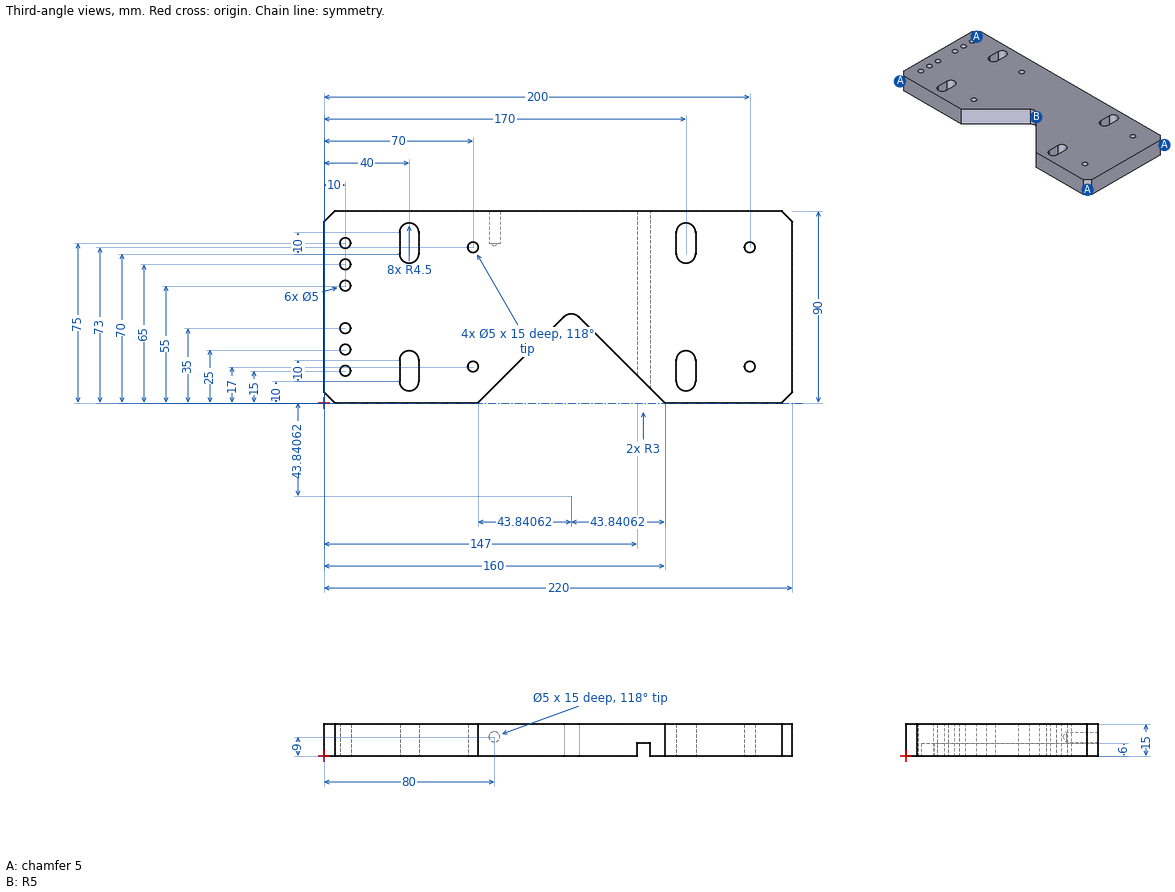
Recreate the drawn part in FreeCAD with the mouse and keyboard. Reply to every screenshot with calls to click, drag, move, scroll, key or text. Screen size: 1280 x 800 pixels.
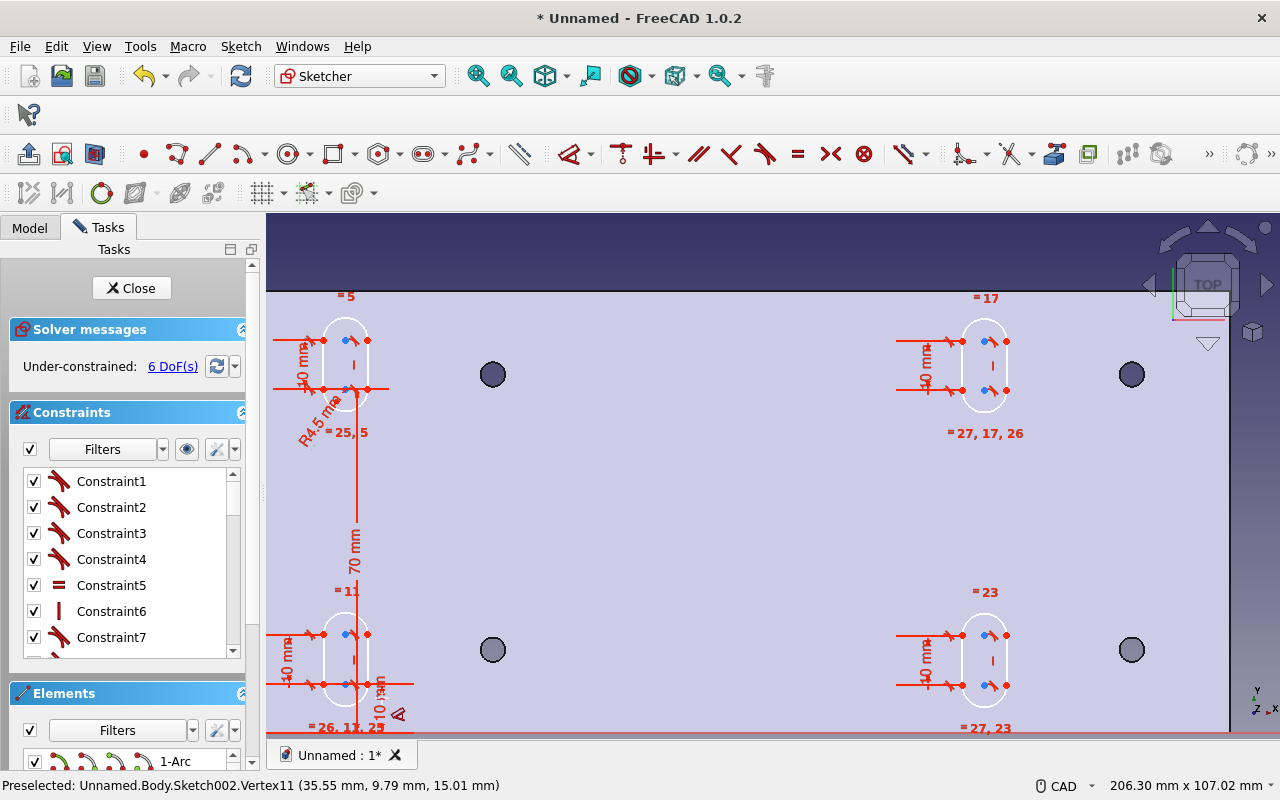
click(962, 390)
click(996, 551)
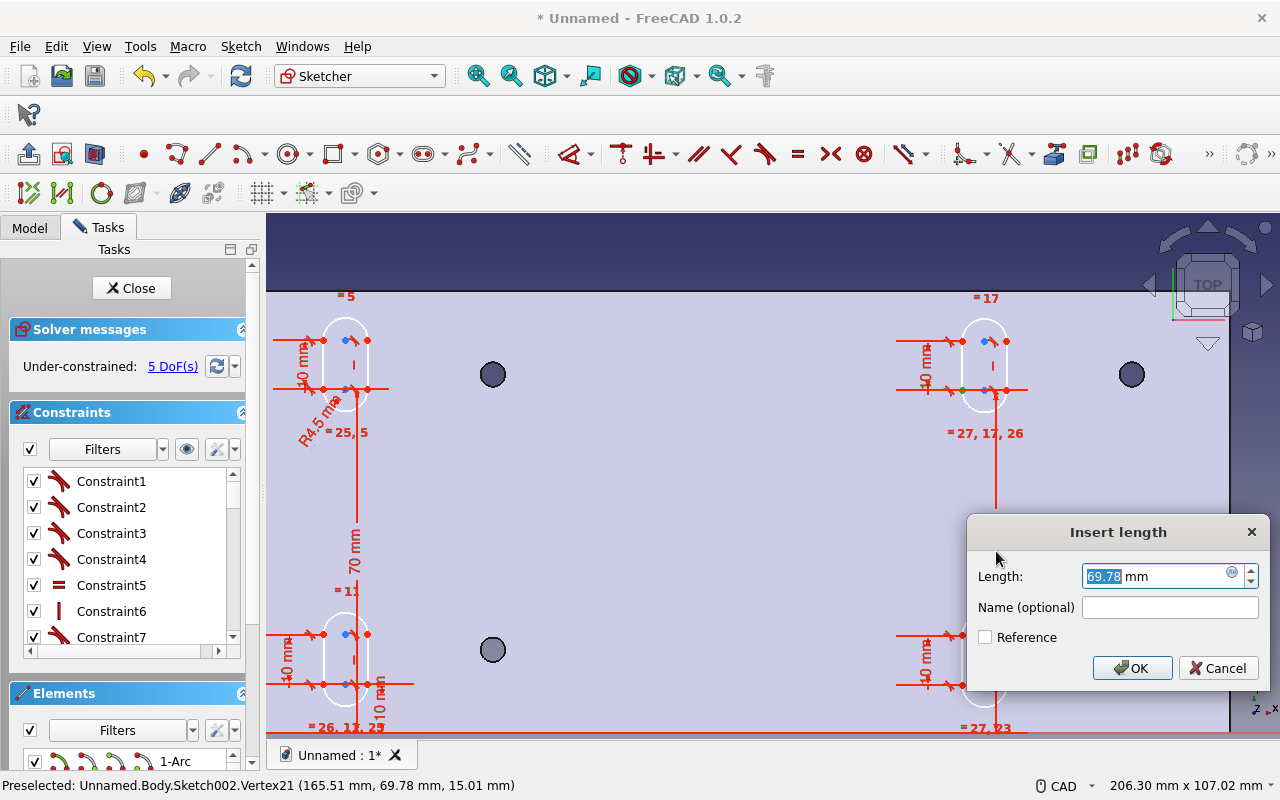
text(70)
key(Return)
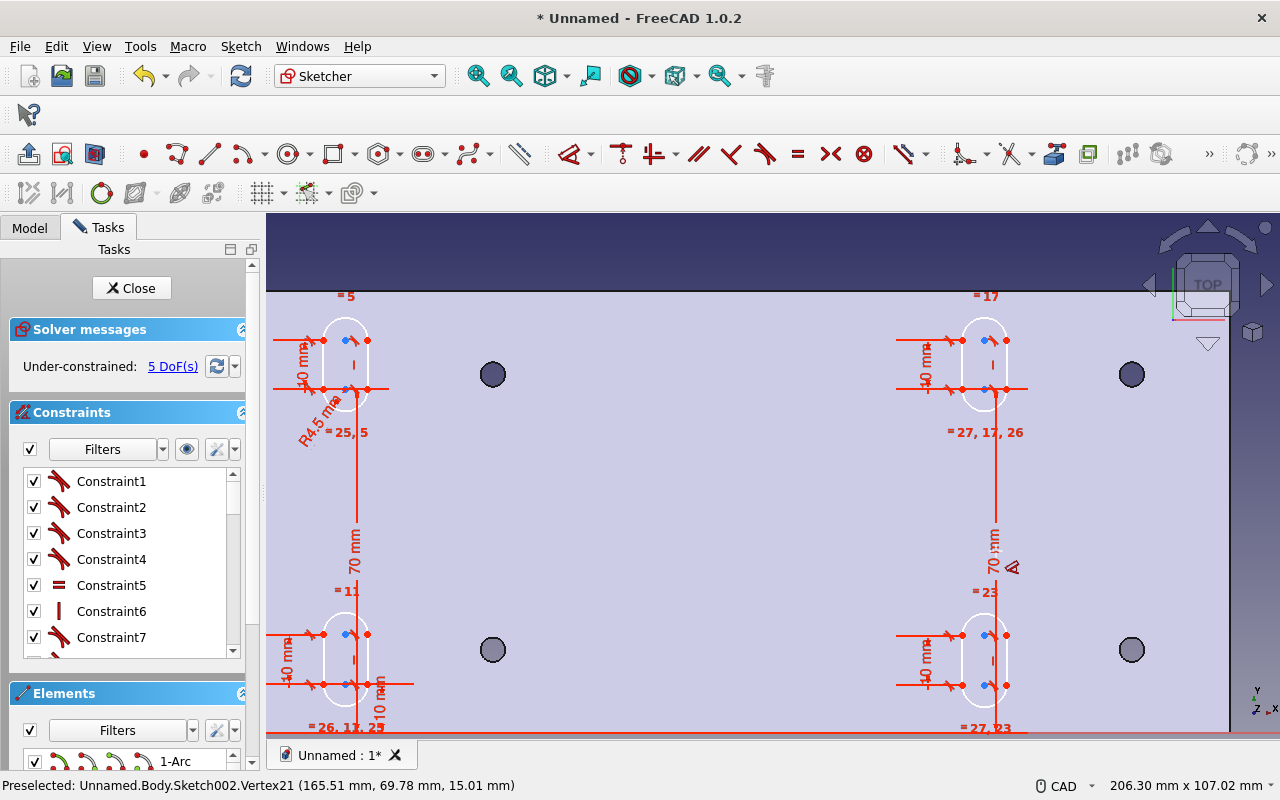
click(962, 685)
click(1020, 698)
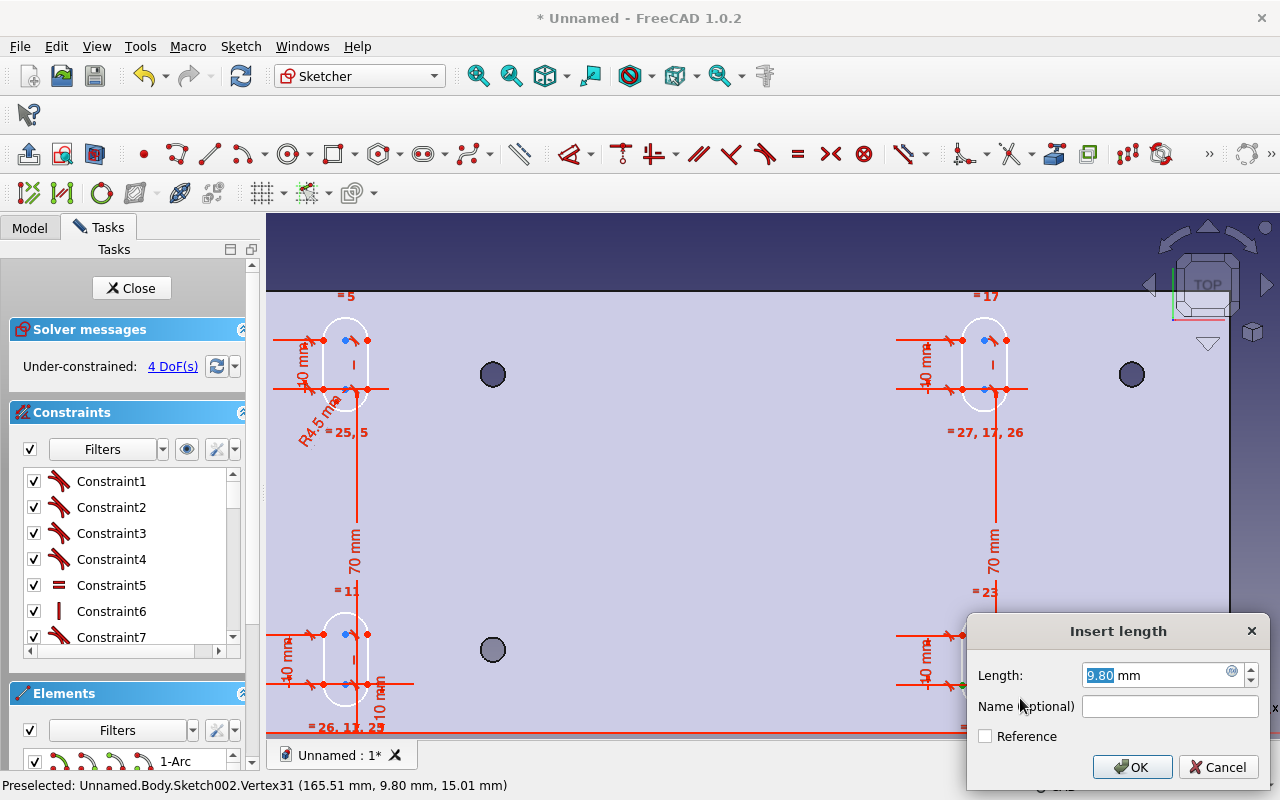
text(10)
key(Return)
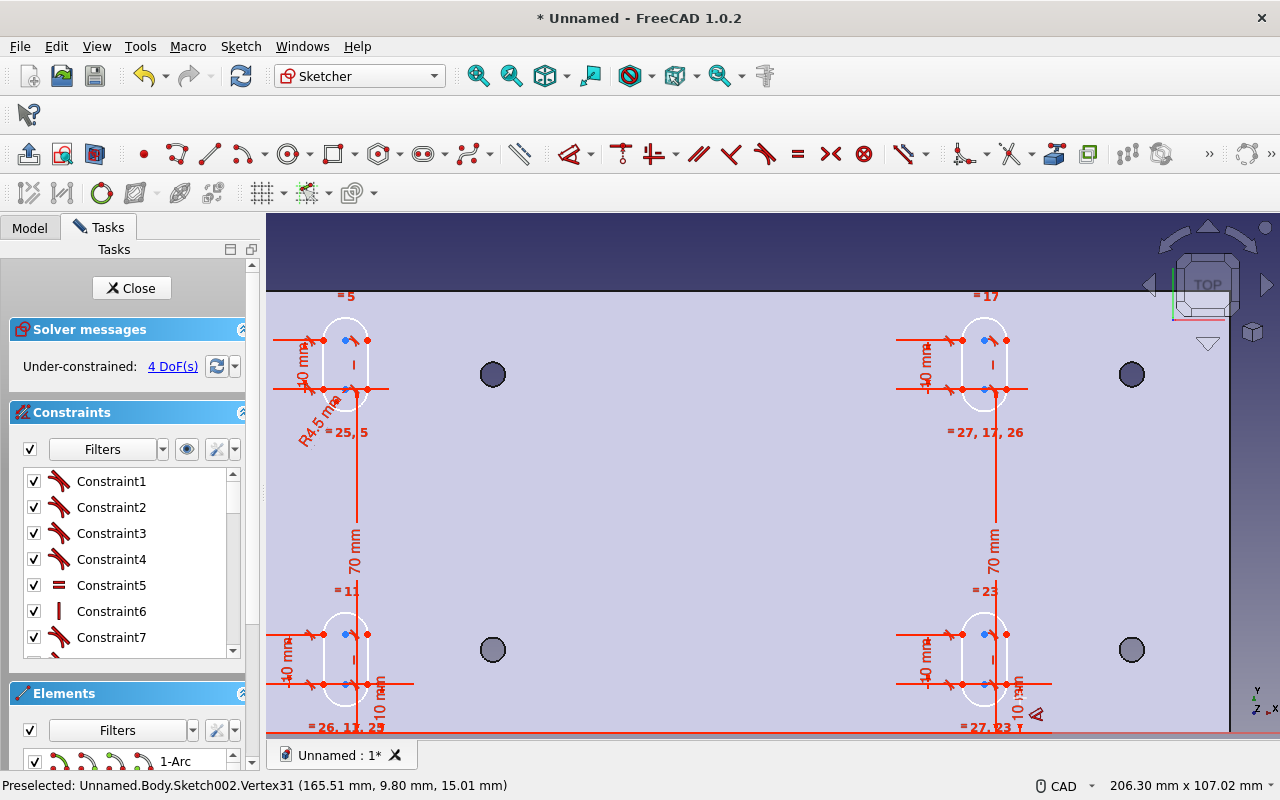
click(346, 389)
click(308, 331)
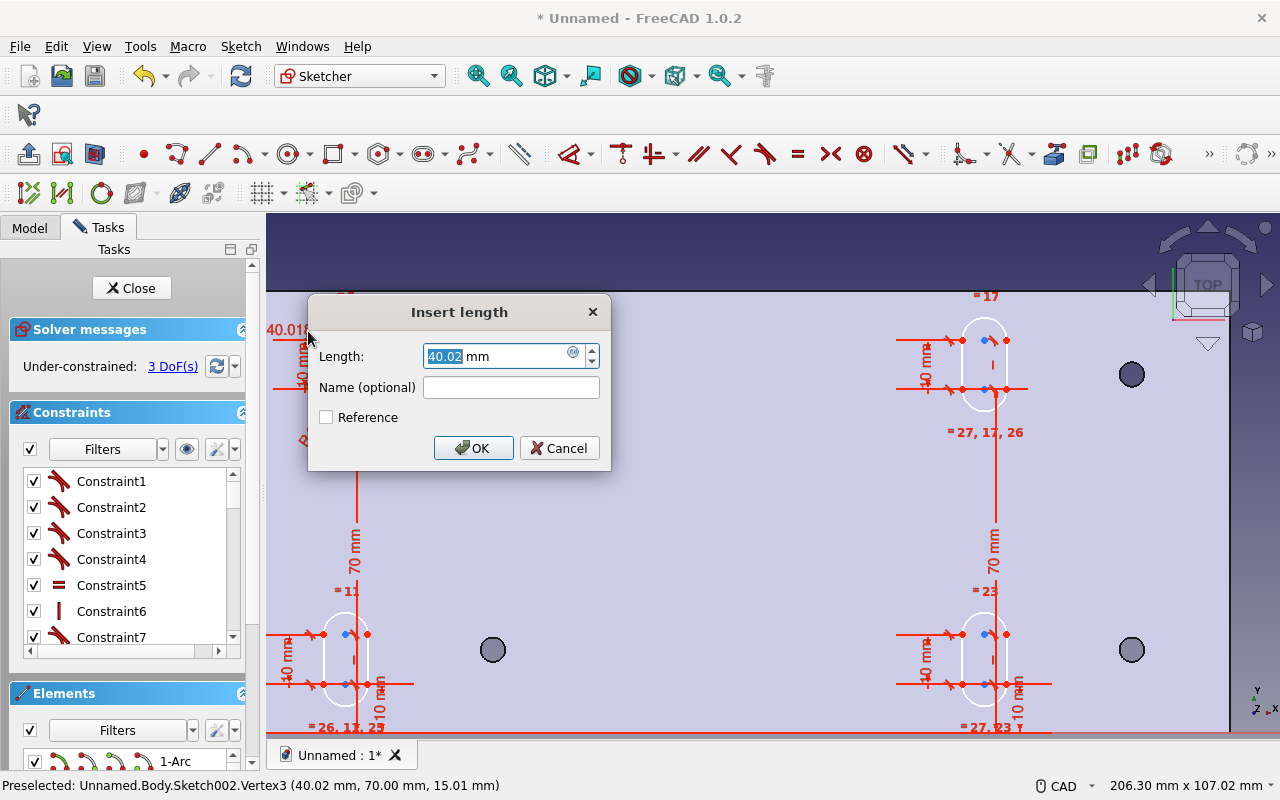
text(40)
key(Return)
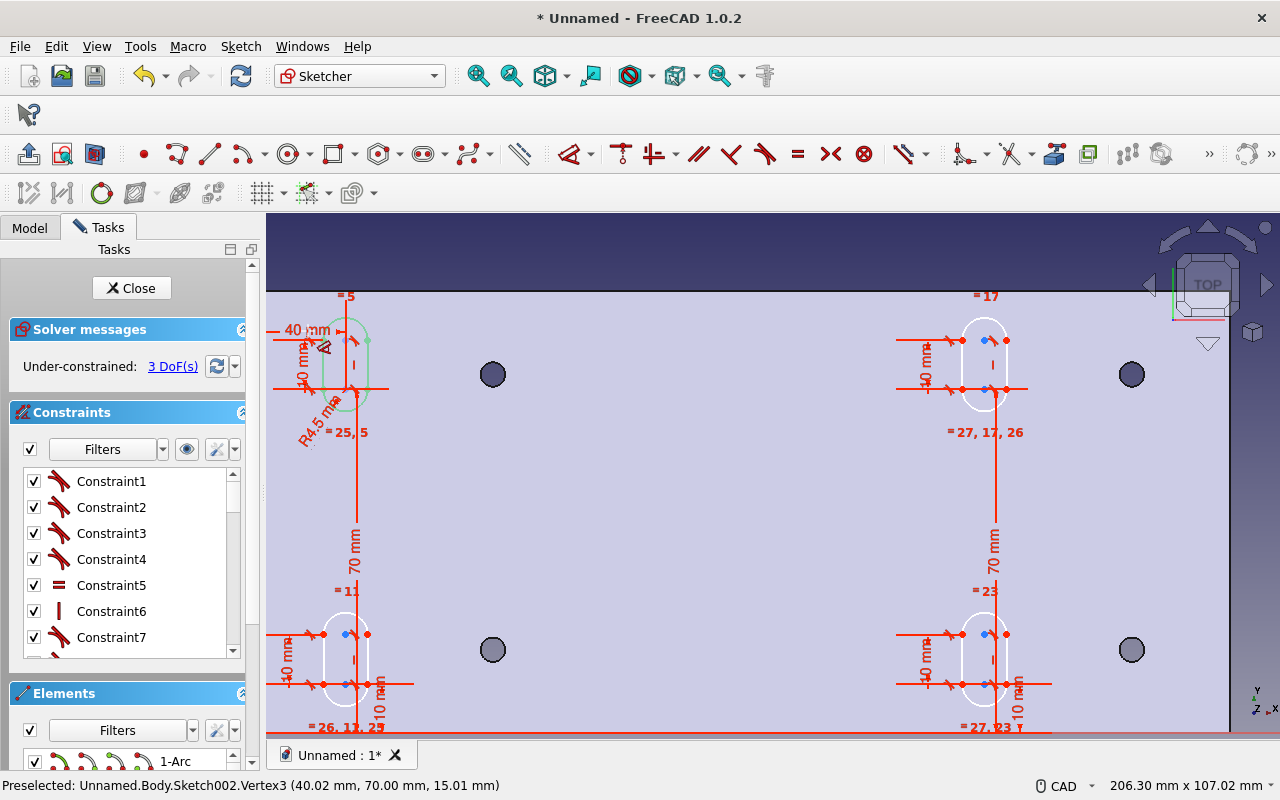
click(346, 684)
click(308, 626)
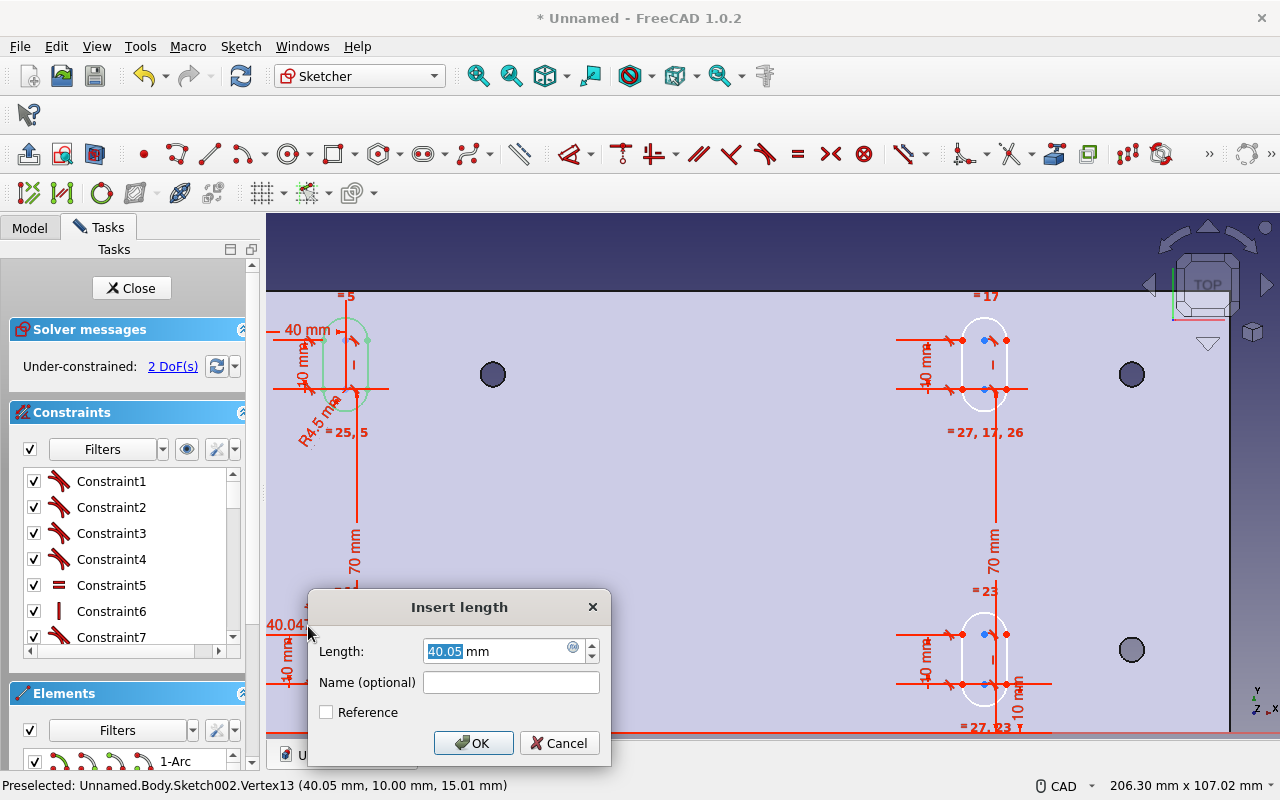
text(40)
key(Return)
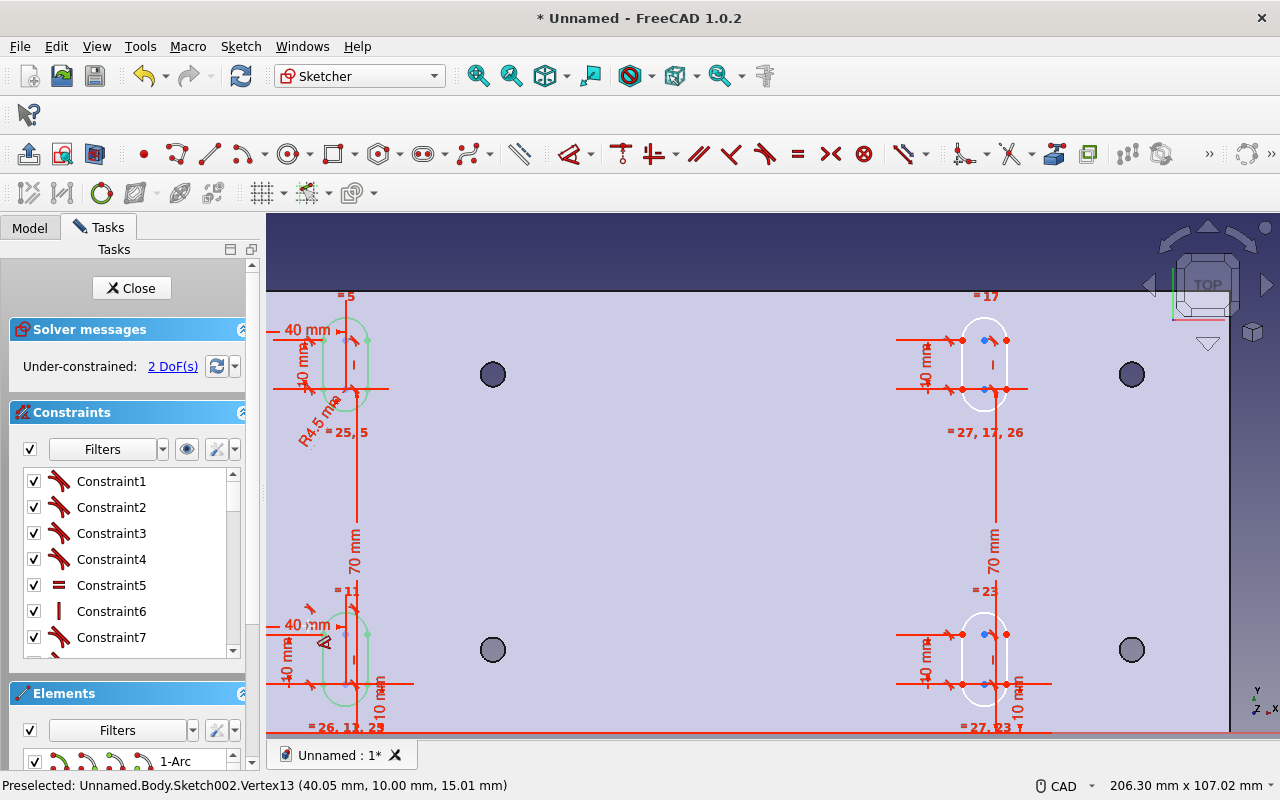
click(984, 389)
click(639, 355)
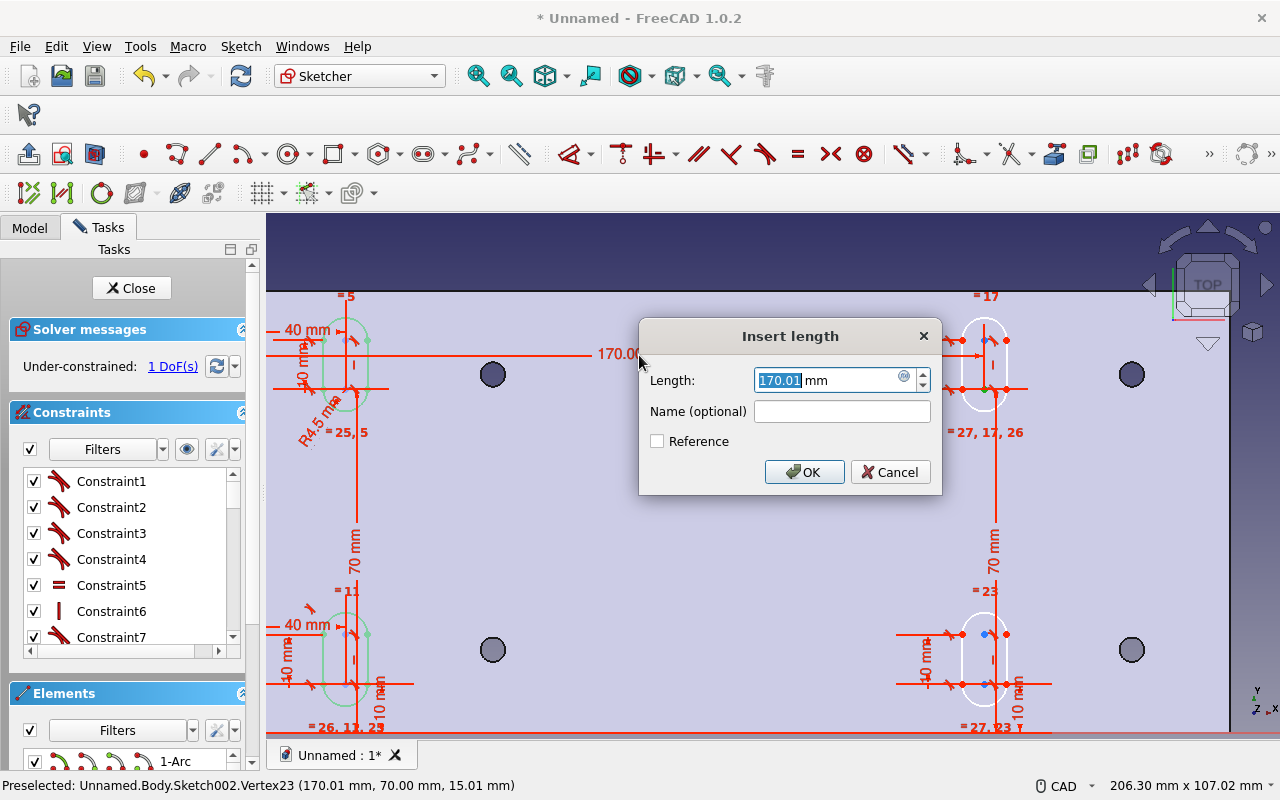
text(170)
key(Return)